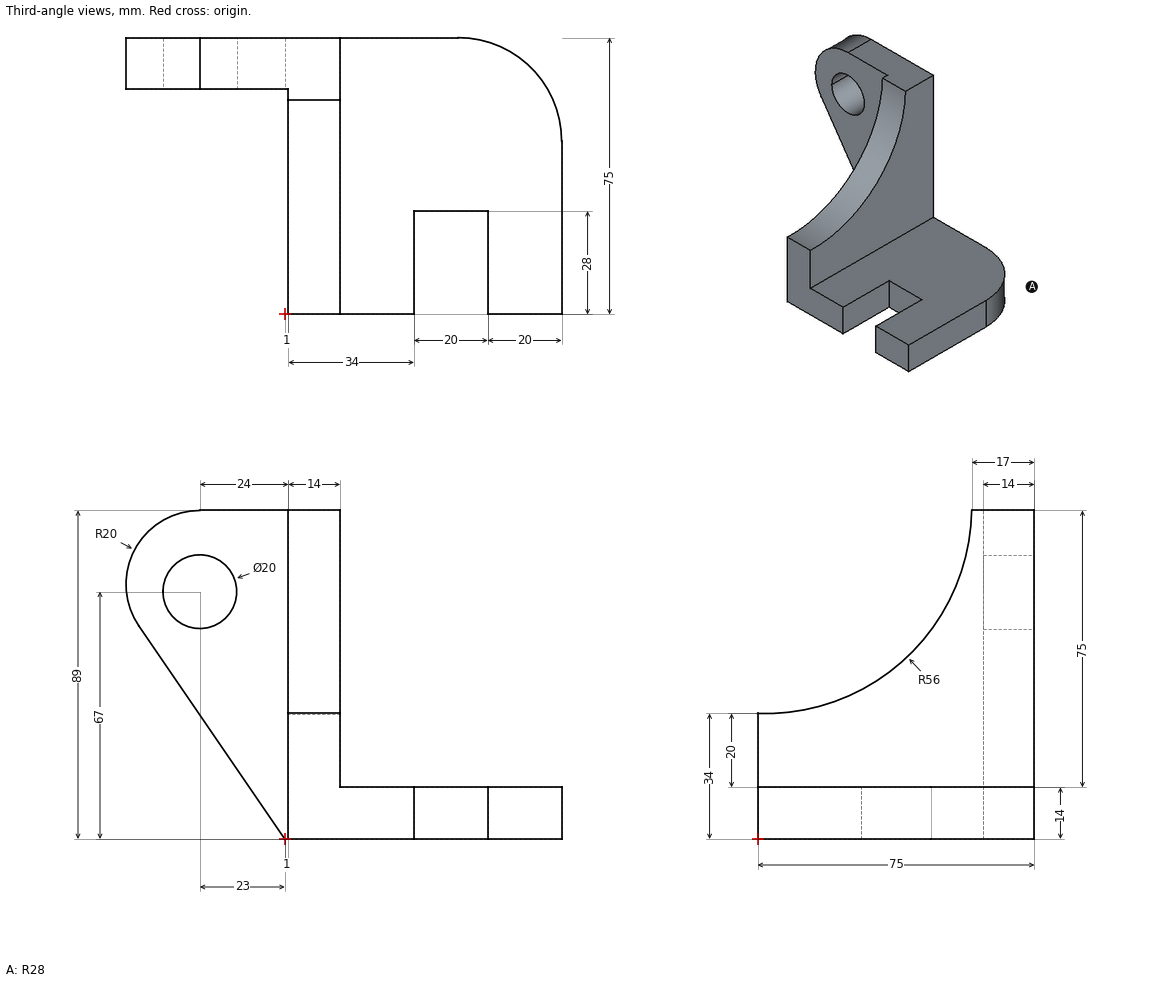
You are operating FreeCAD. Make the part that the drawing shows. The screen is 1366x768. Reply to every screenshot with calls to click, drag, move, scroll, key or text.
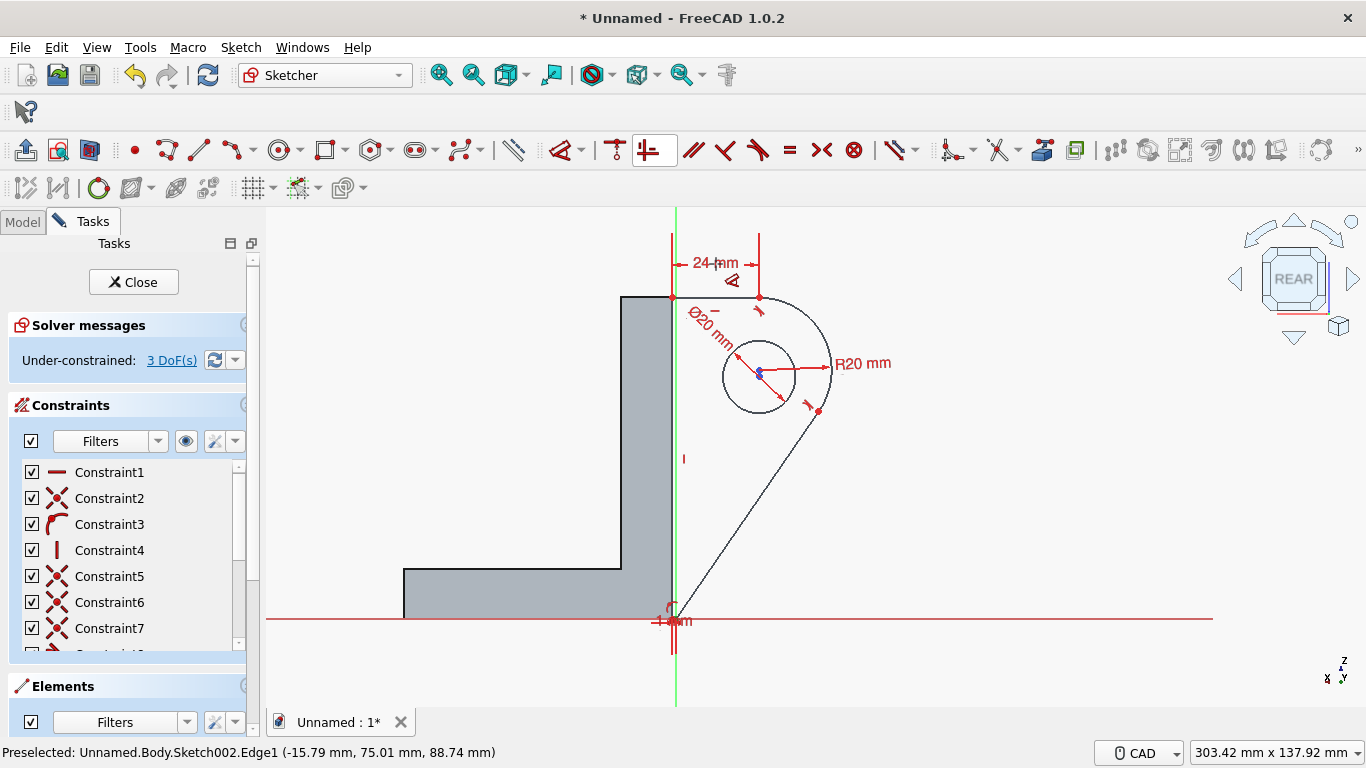
click(672, 394)
click(638, 459)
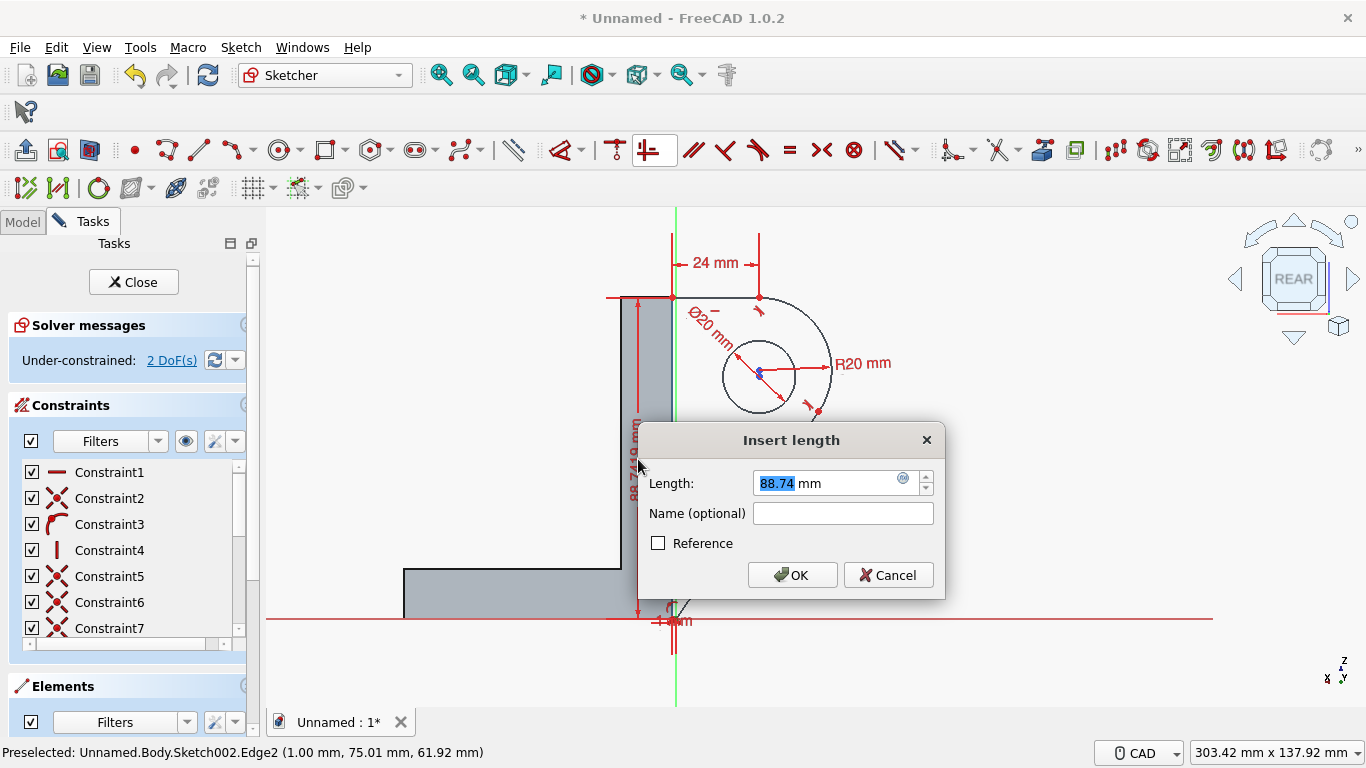
text(89)
key(Return)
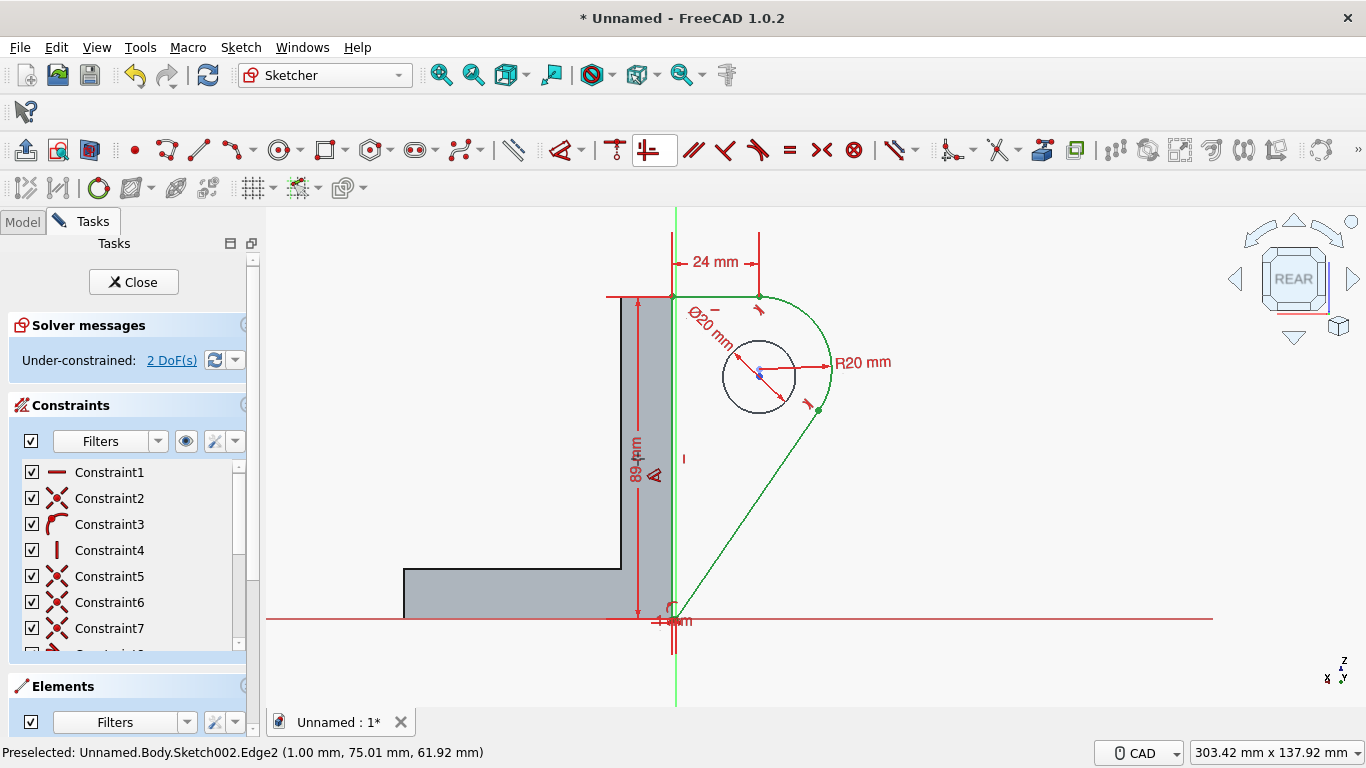
scroll(759, 377, up, 3)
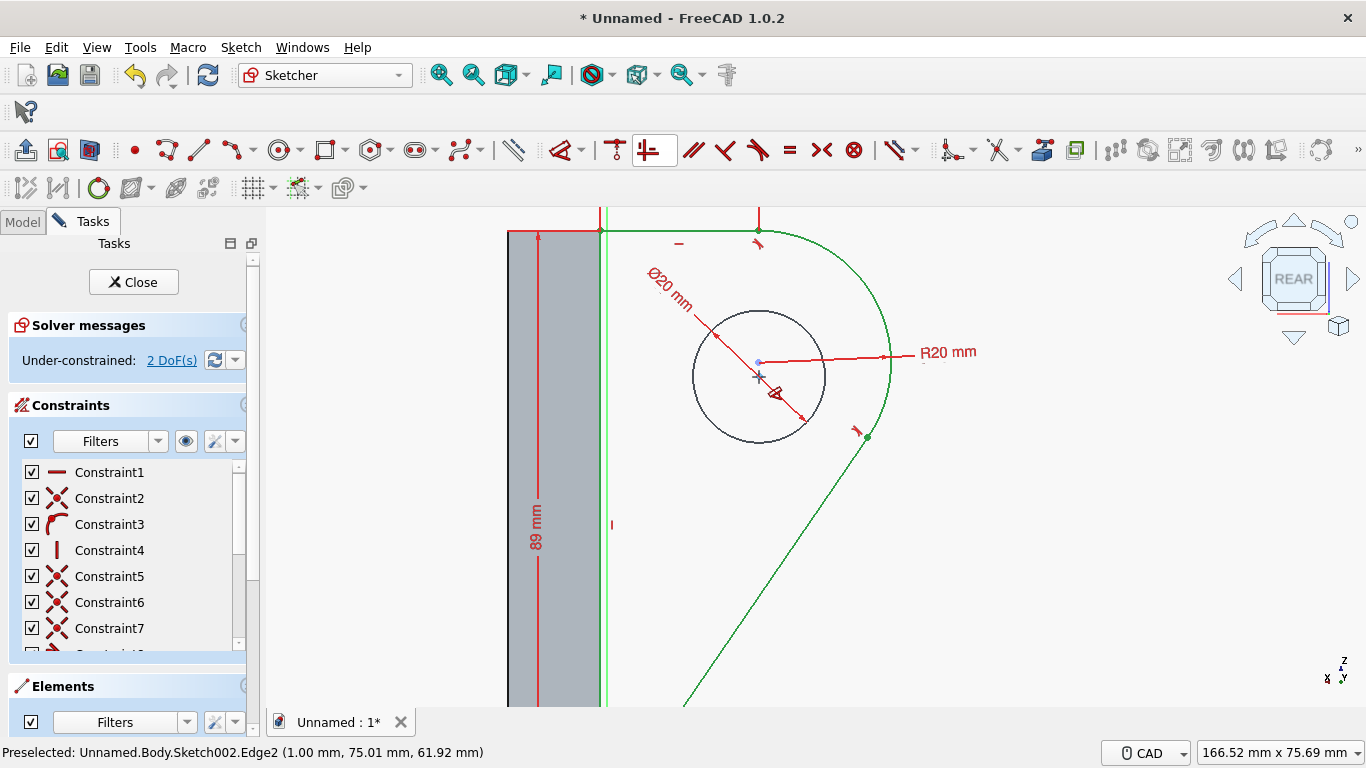
click(759, 377)
click(683, 343)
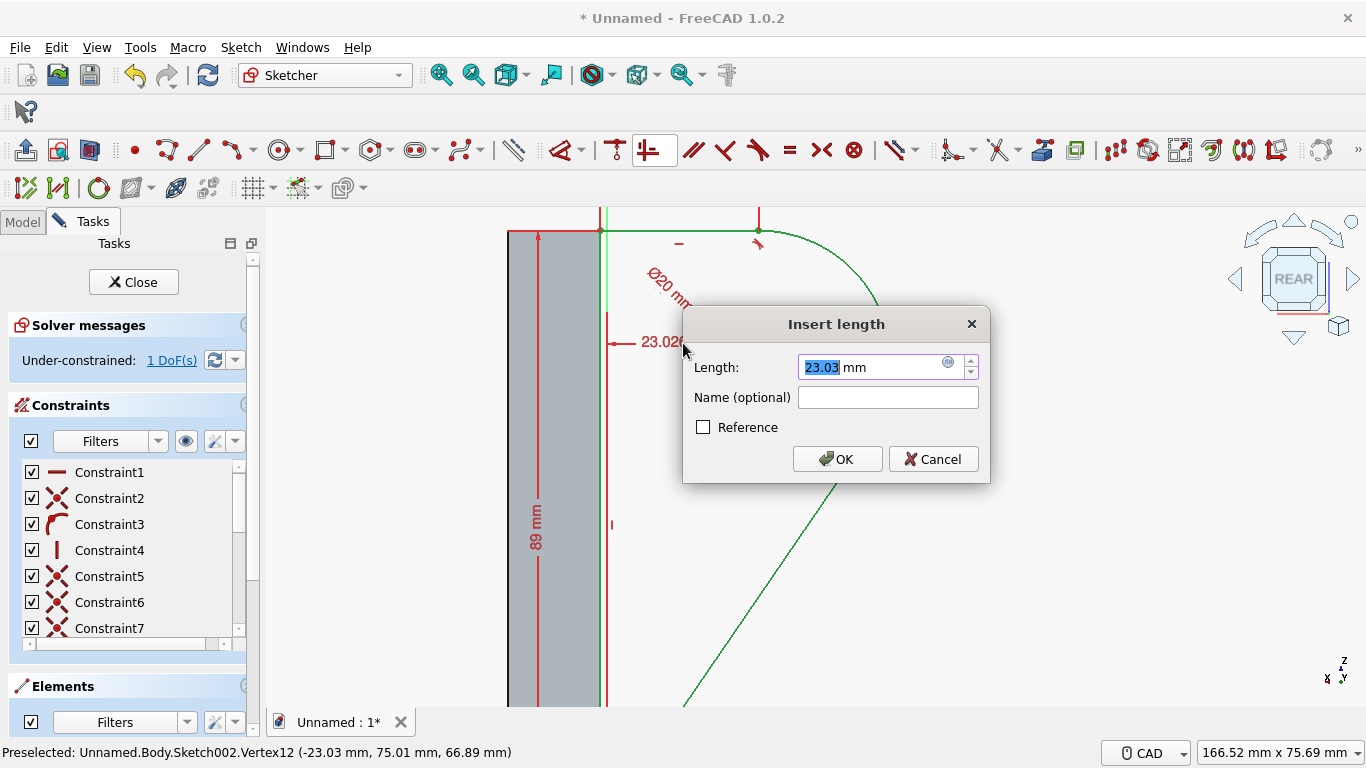
text(23)
key(Return)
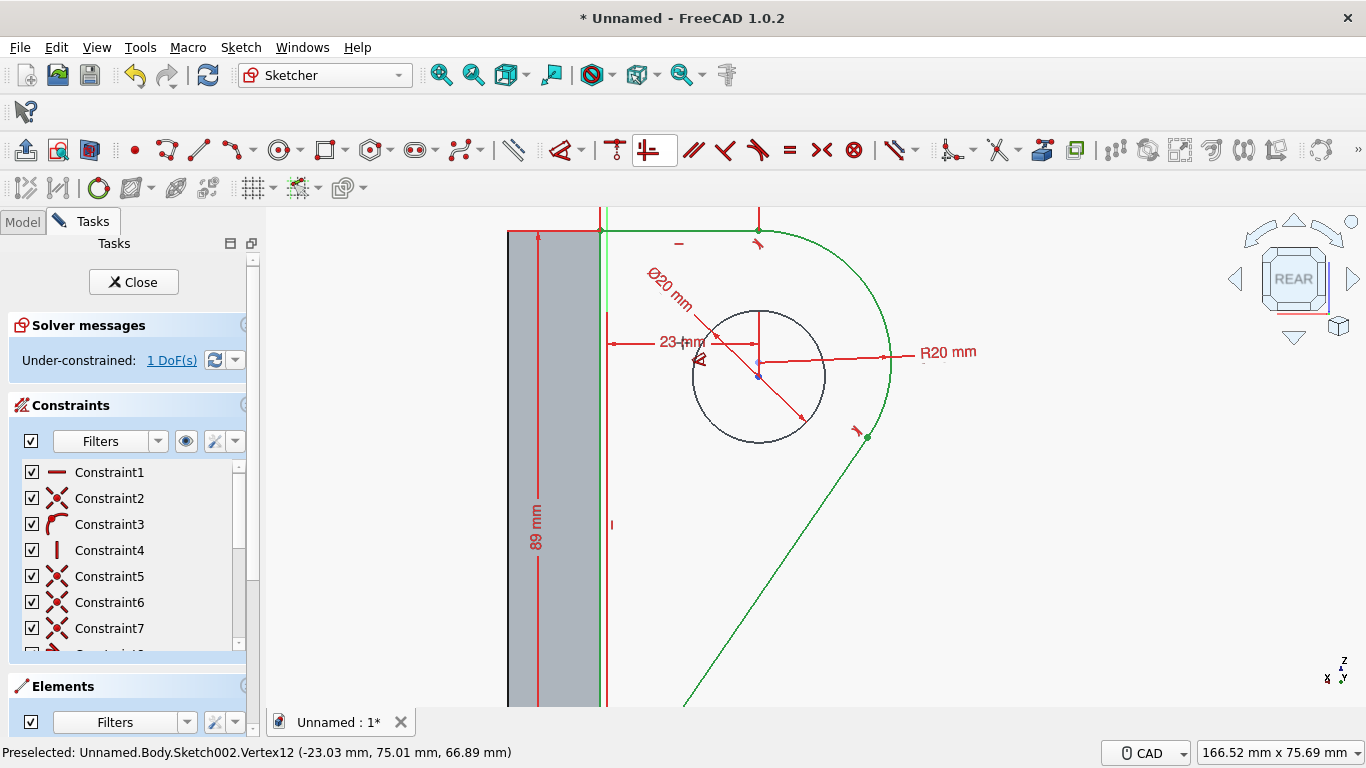
click(759, 377)
click(573, 458)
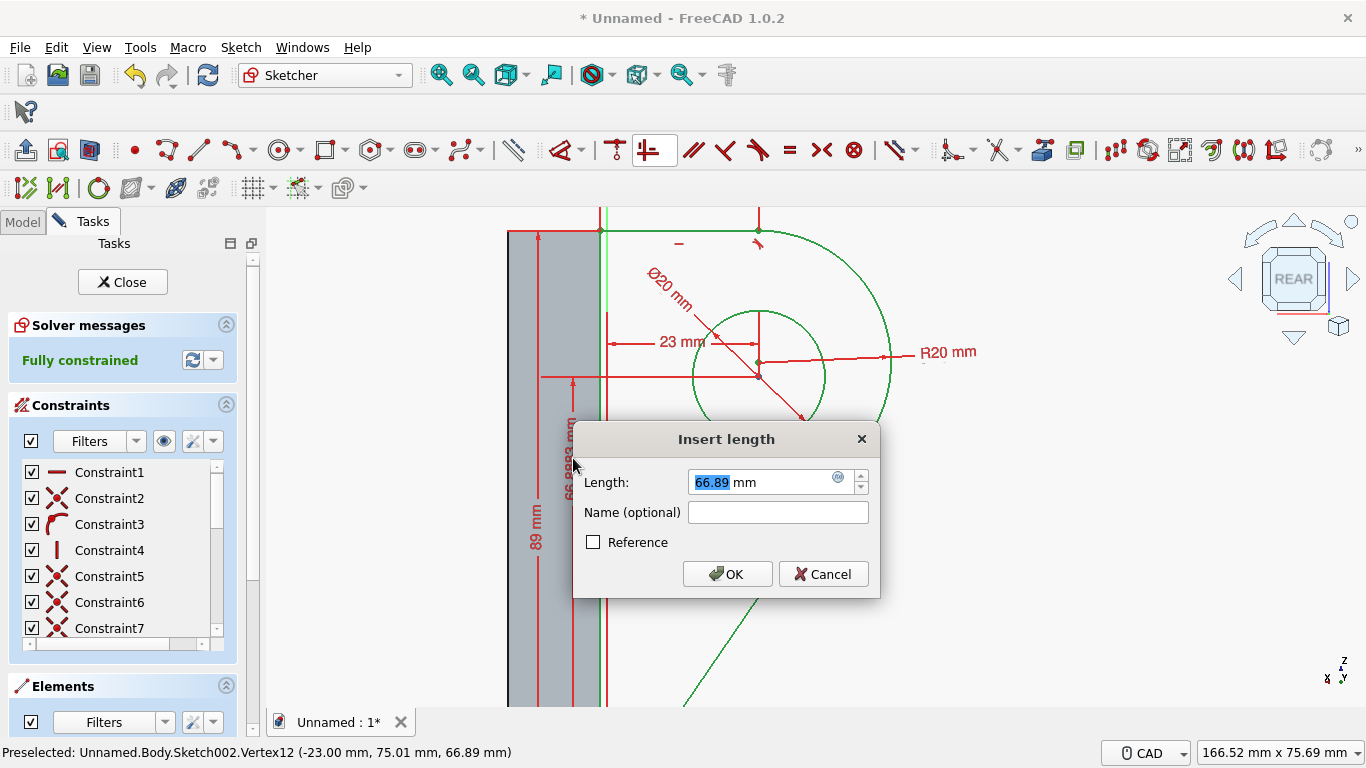
text(67)
key(Return)
key(Escape)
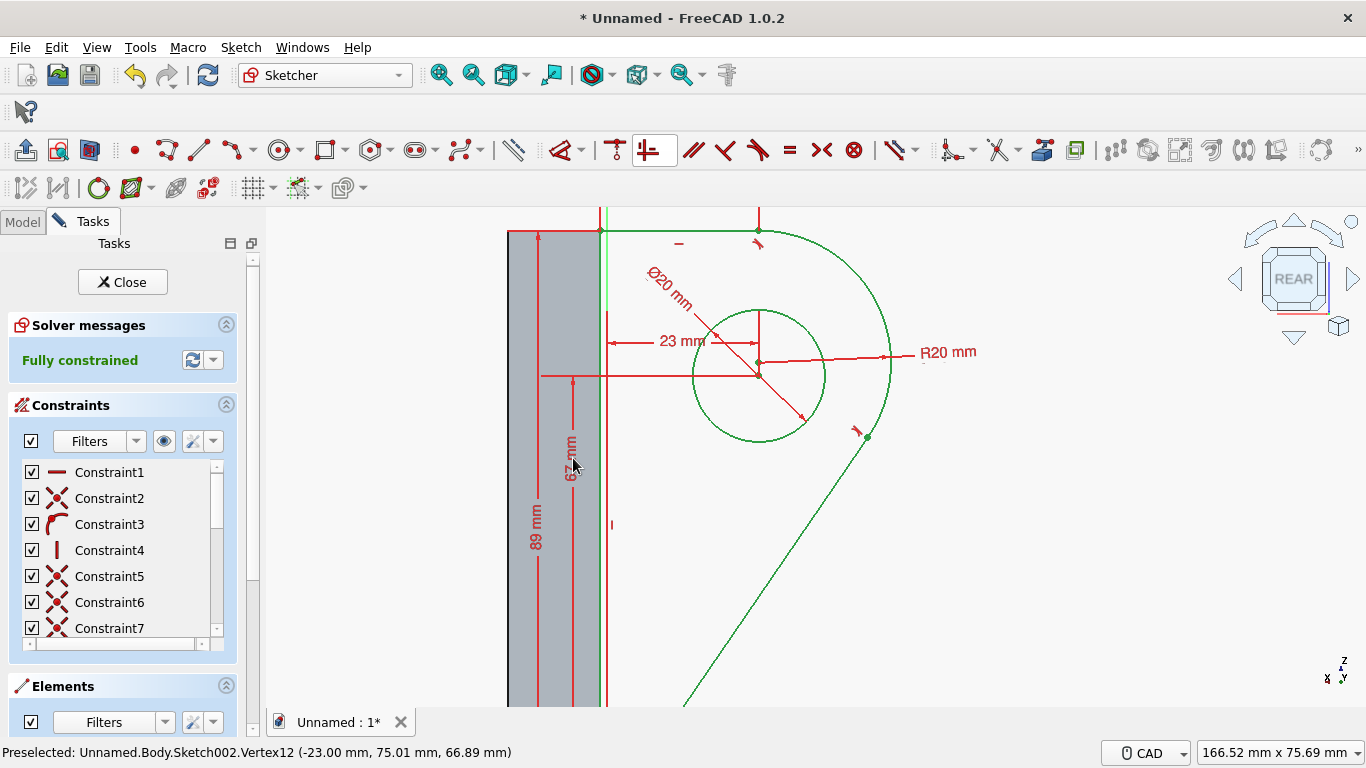
click(123, 282)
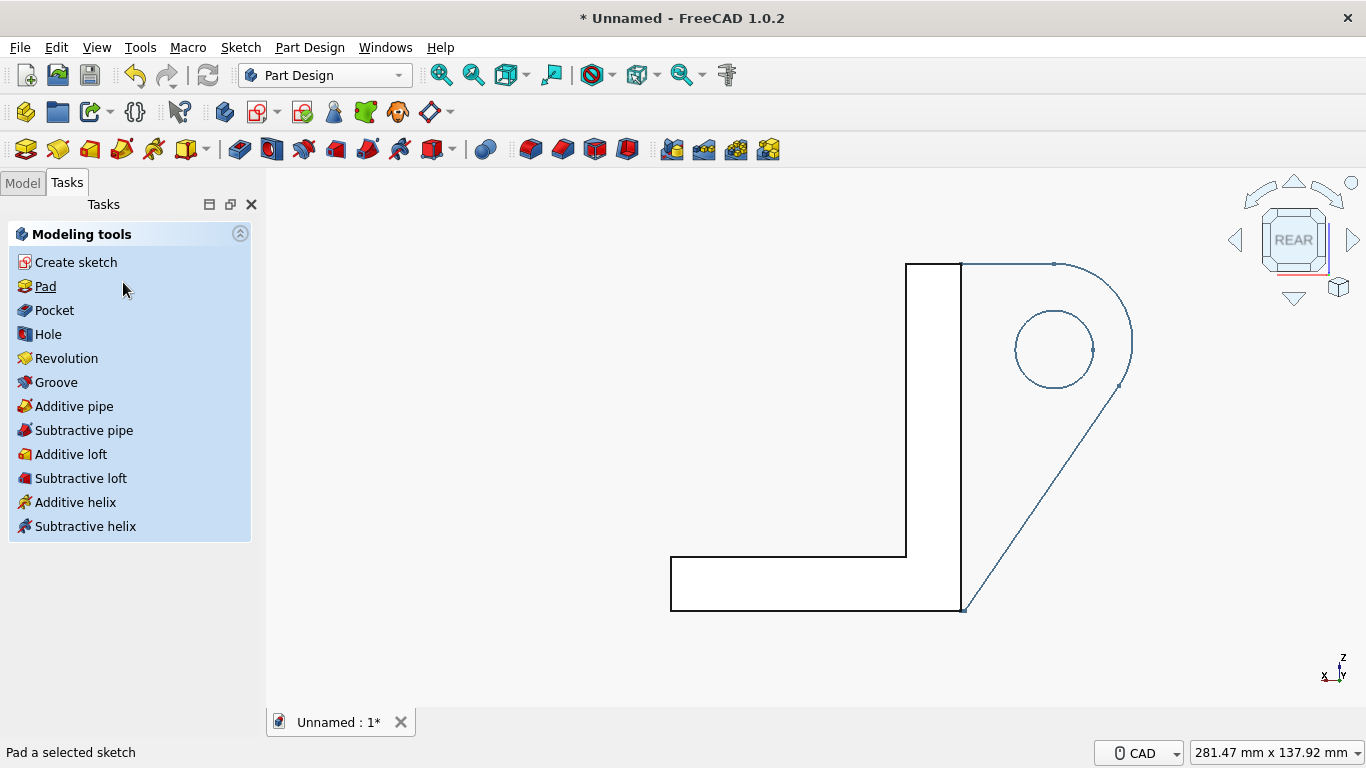
click(26, 150)